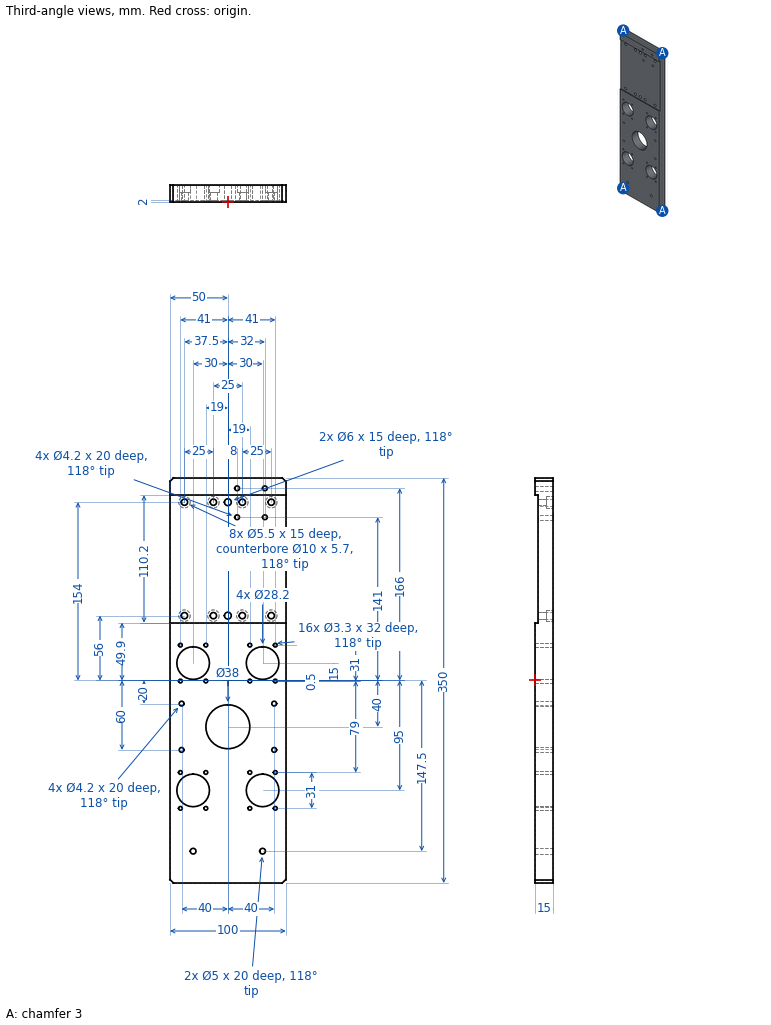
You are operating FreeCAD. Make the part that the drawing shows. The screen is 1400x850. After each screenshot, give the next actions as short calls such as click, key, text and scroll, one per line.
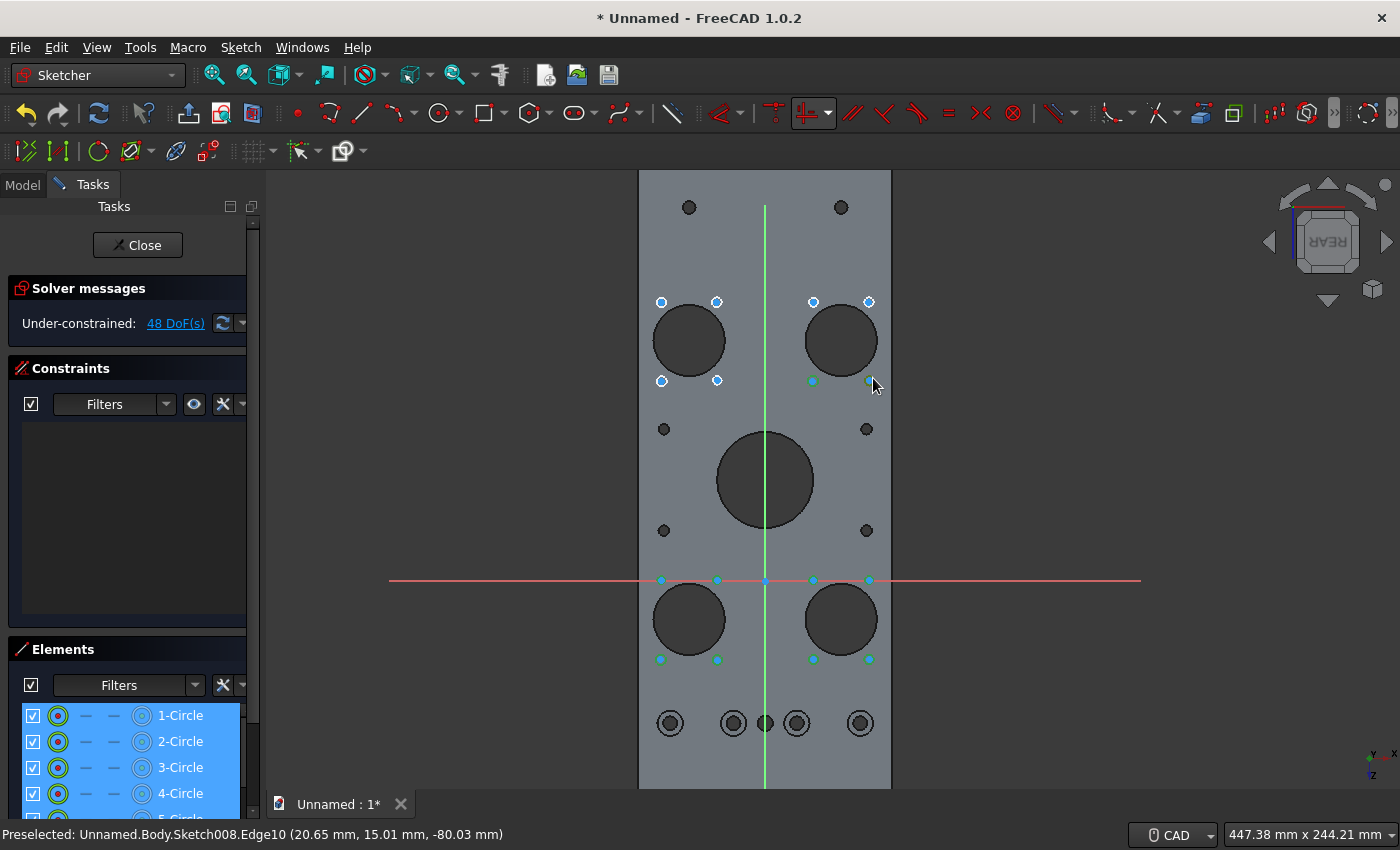
scroll(872, 299, up, 6)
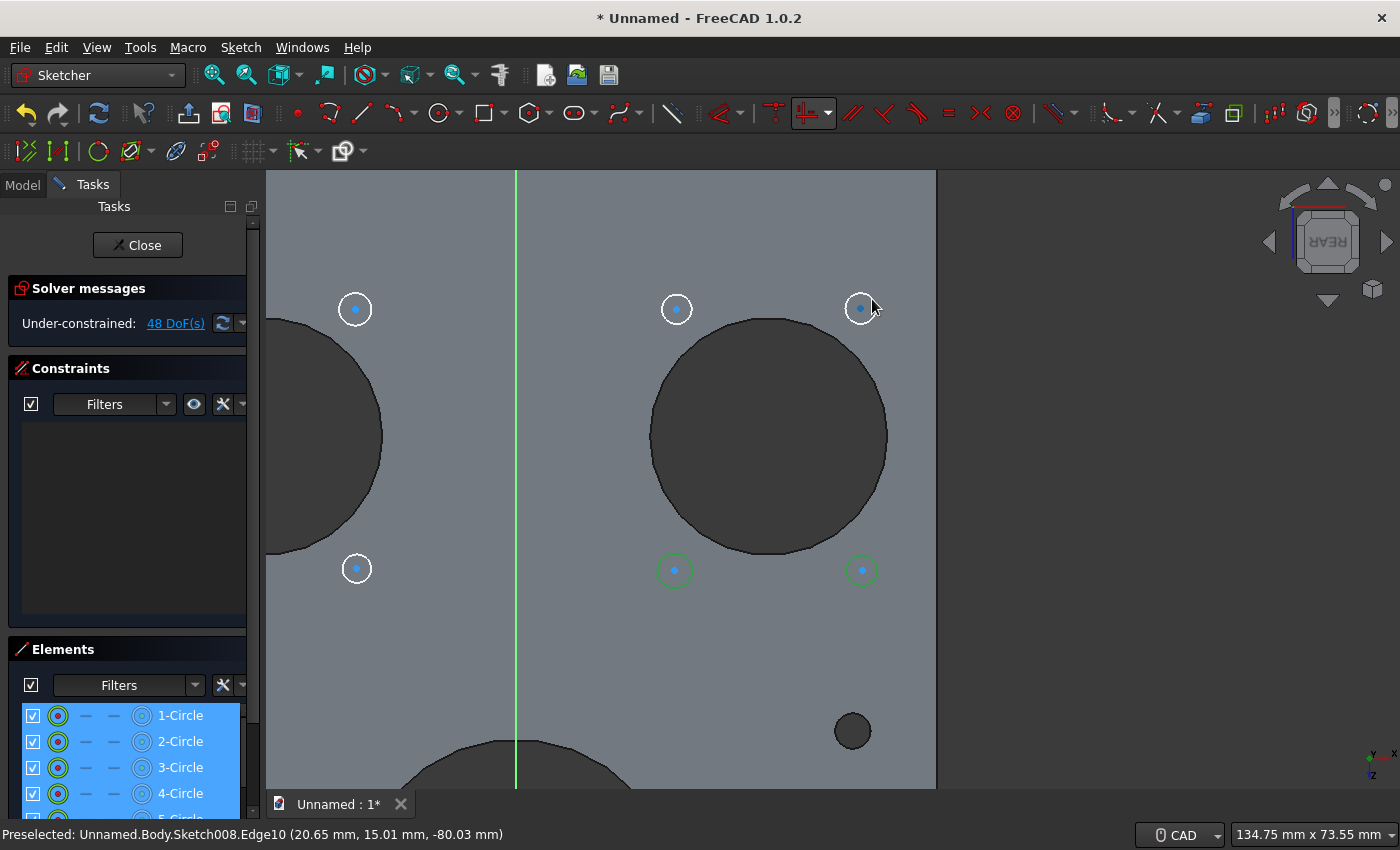
click(872, 298)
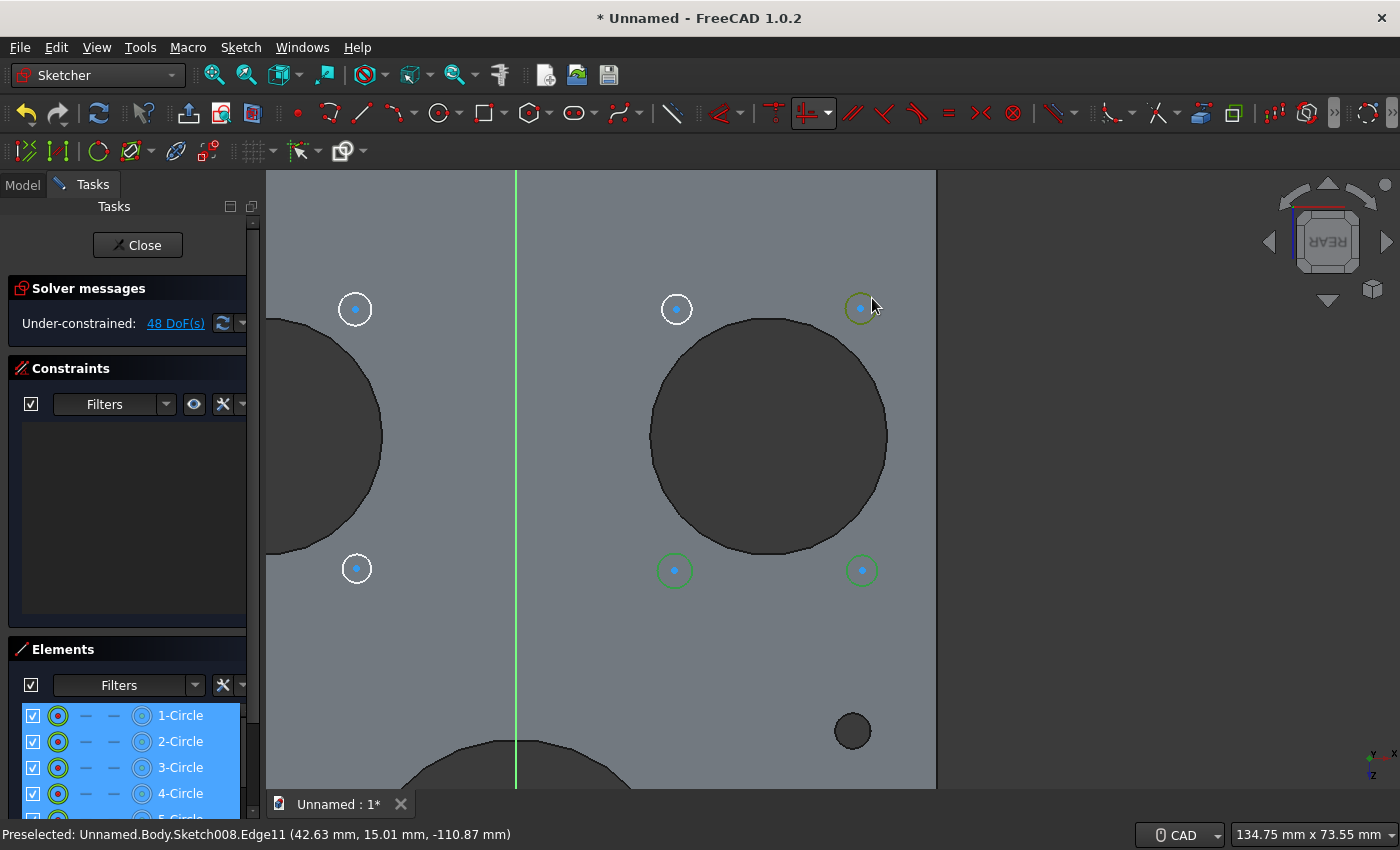
click(687, 299)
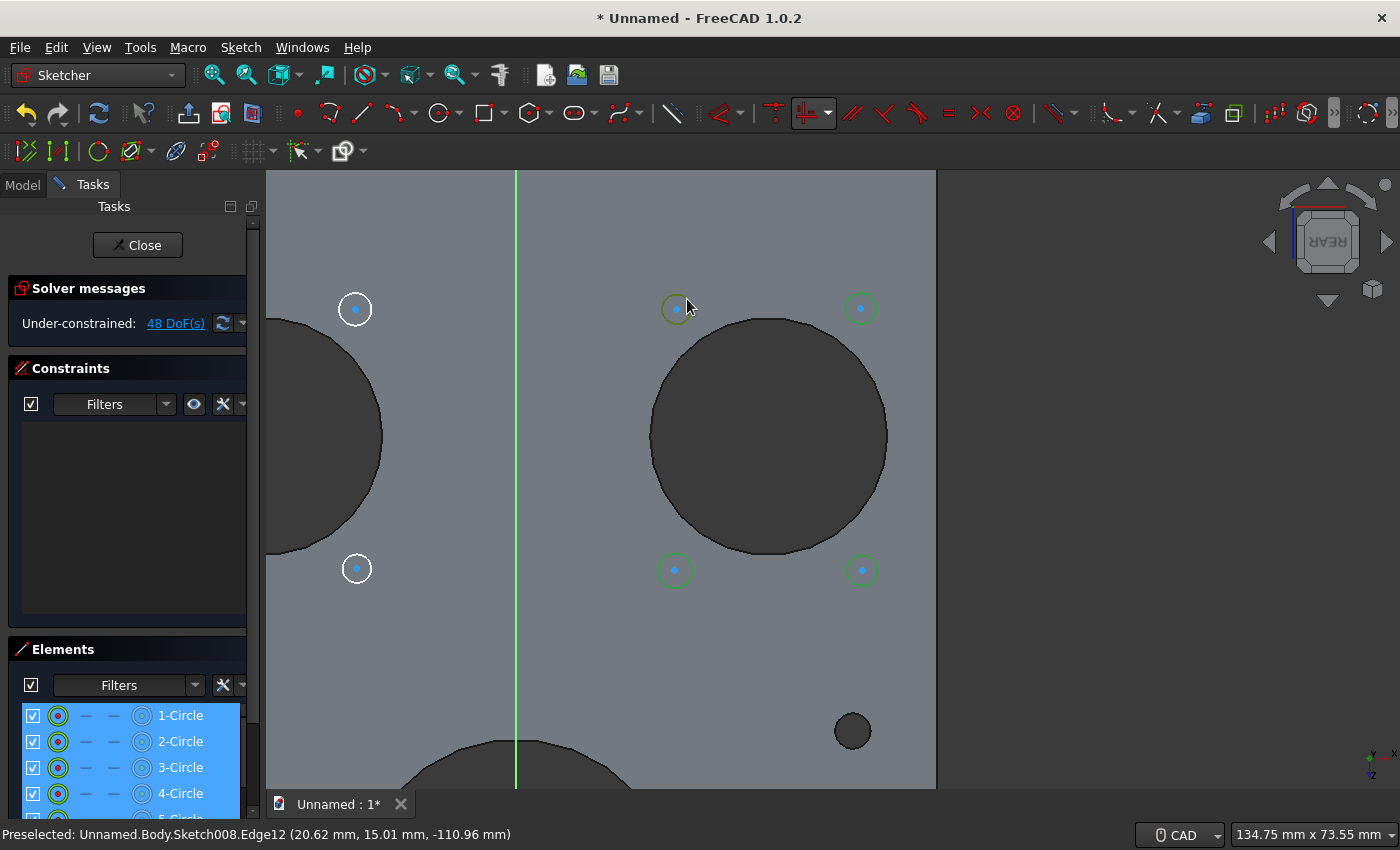
click(367, 559)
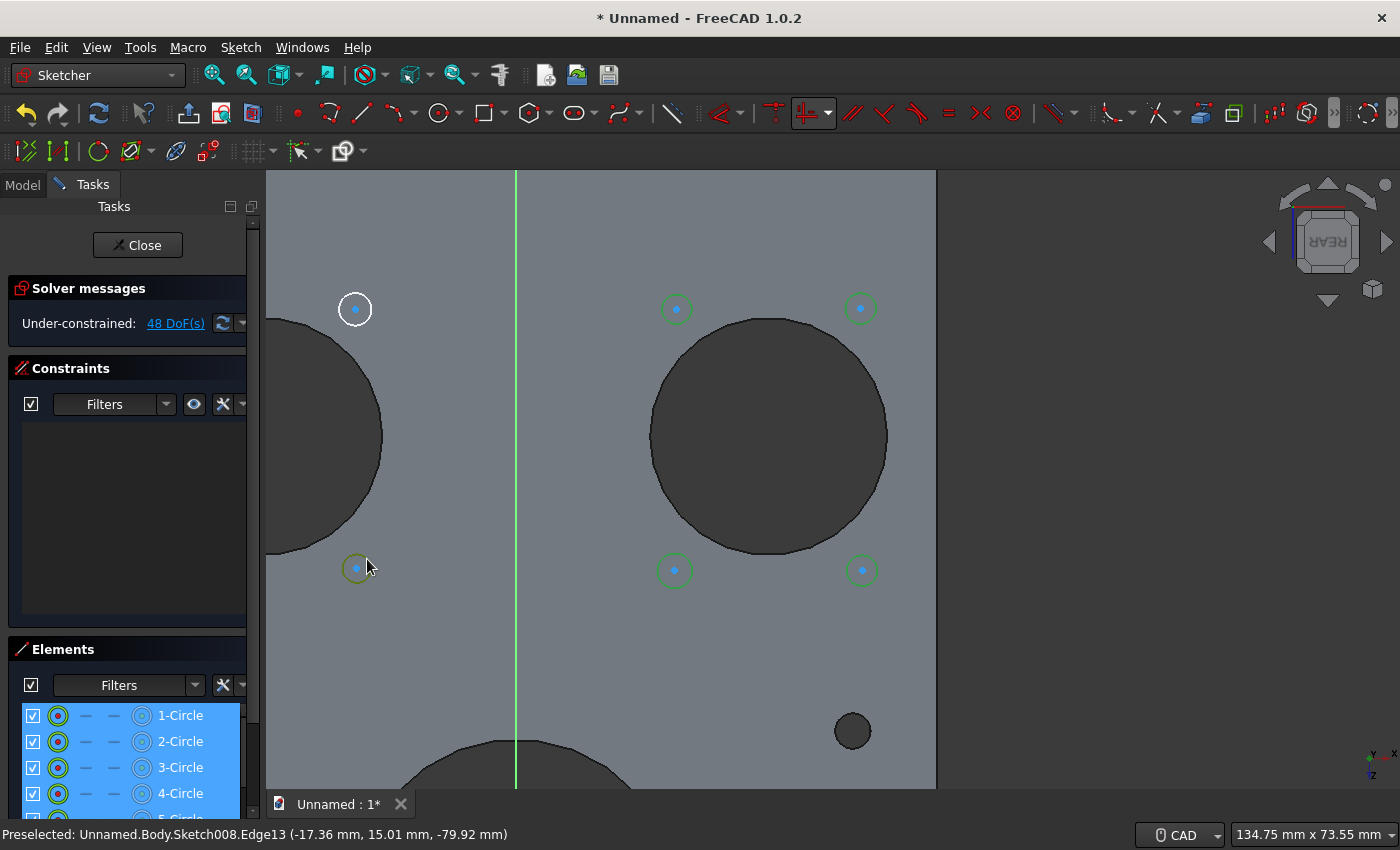
scroll(872, 299, down, 6)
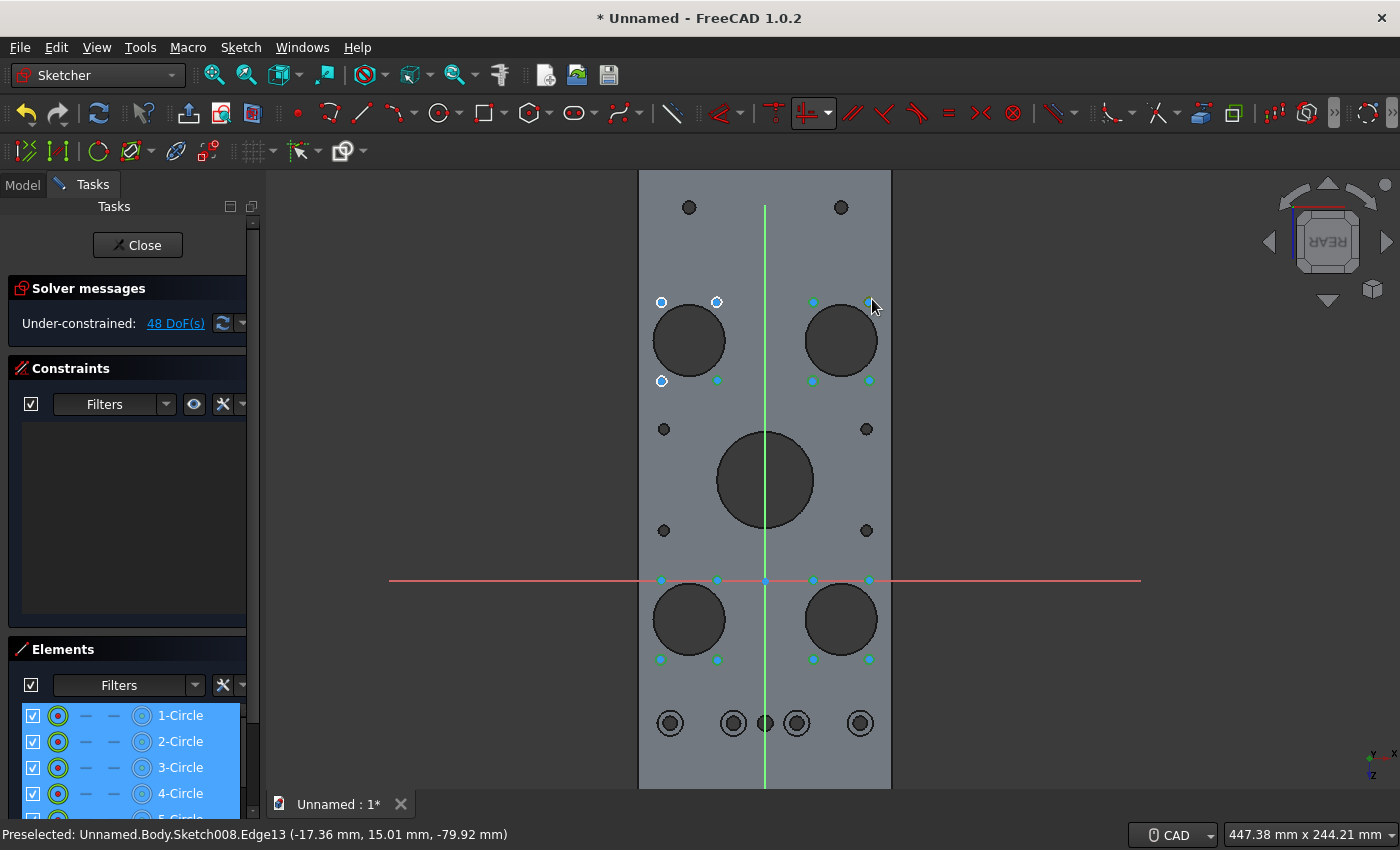
scroll(665, 378, up, 6)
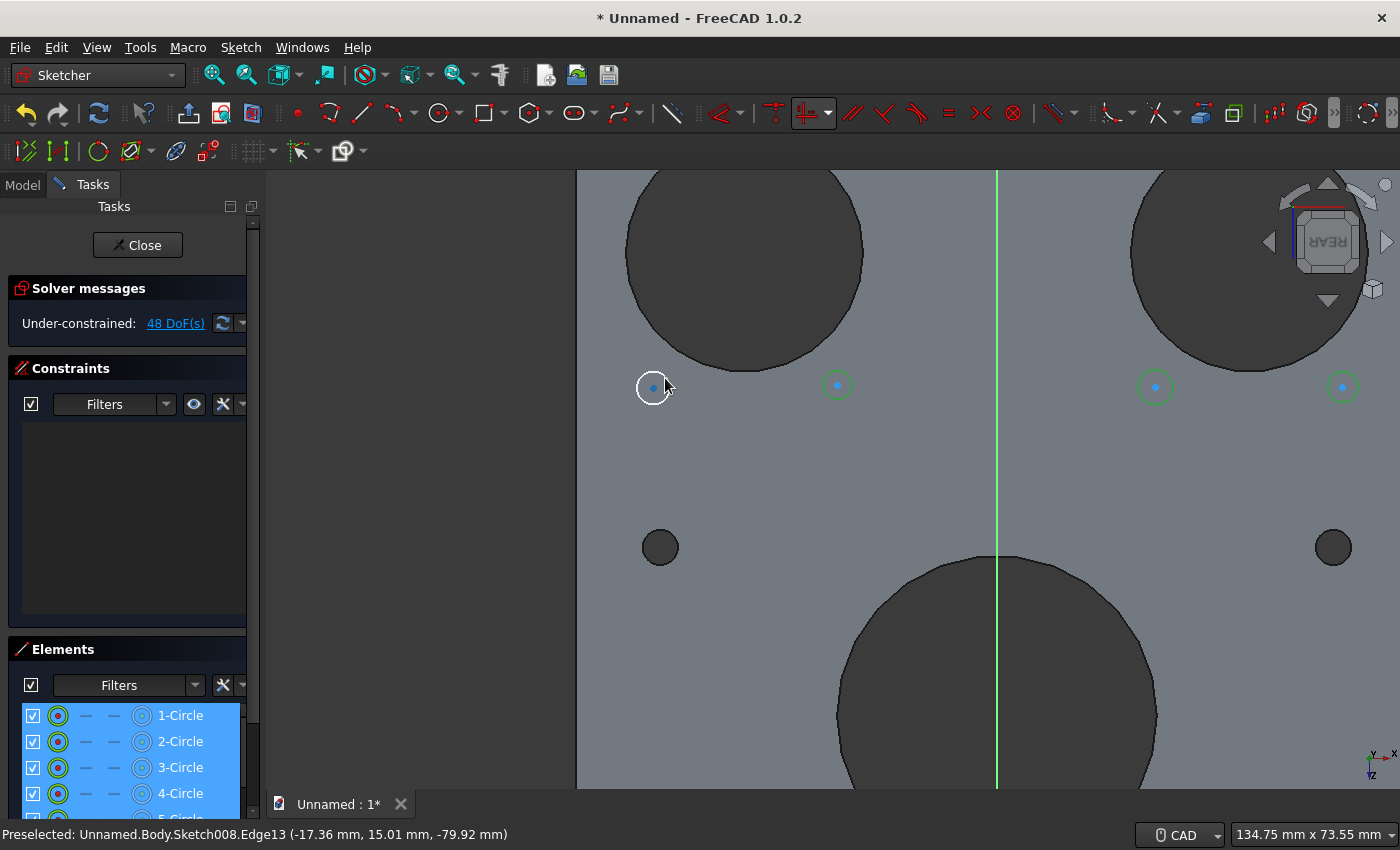
click(665, 376)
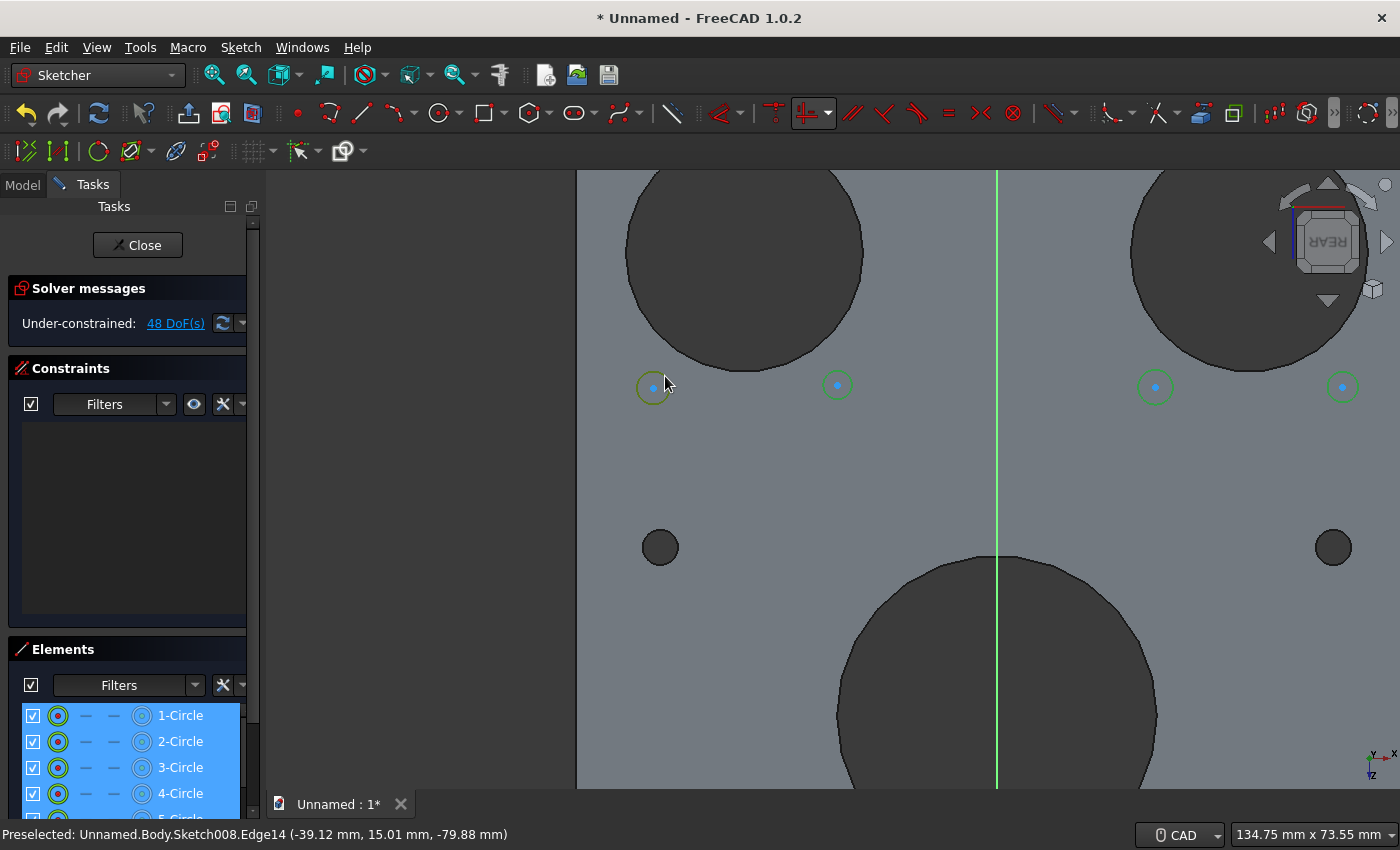
scroll(664, 378, down, 6)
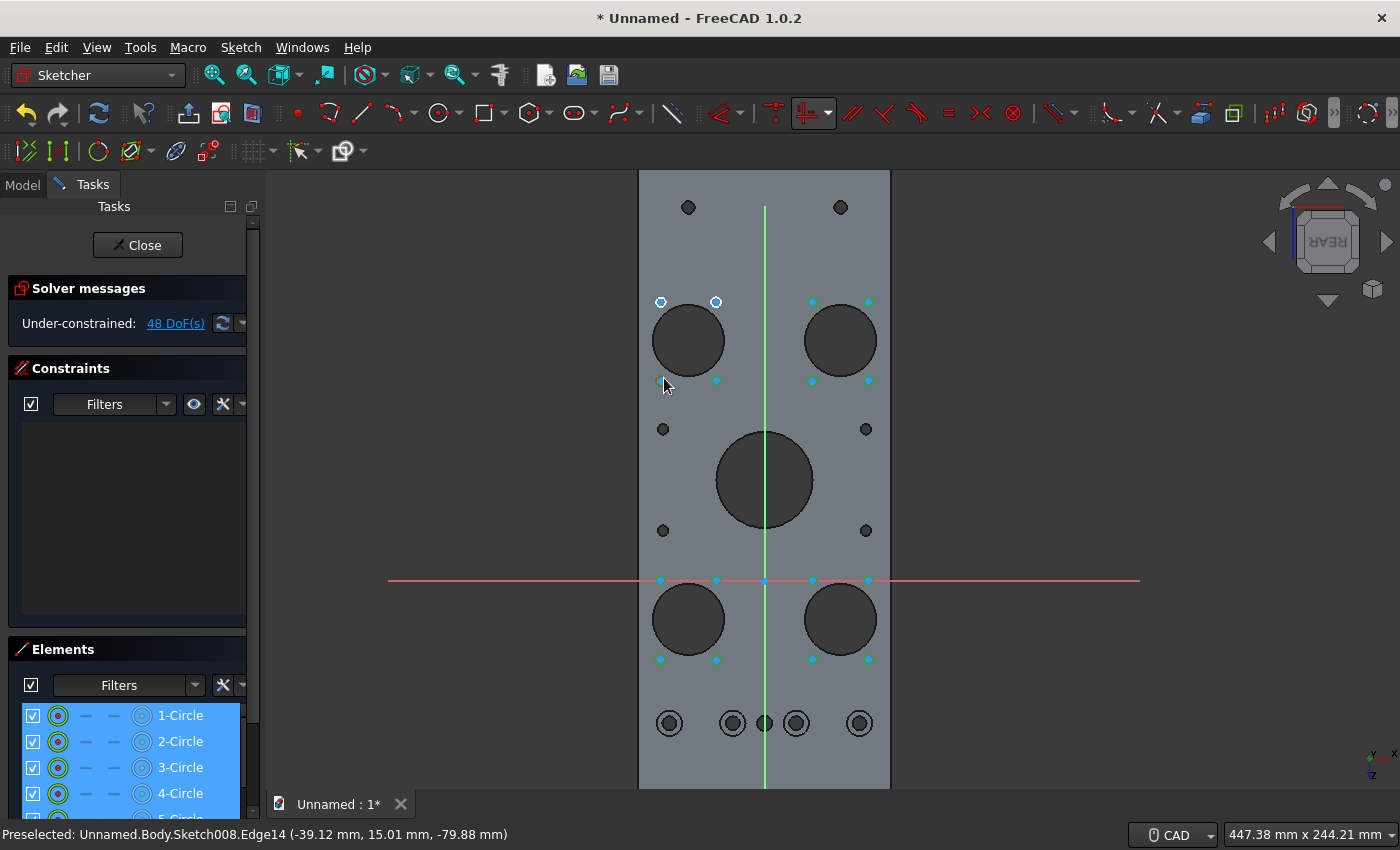
scroll(719, 299, up, 6)